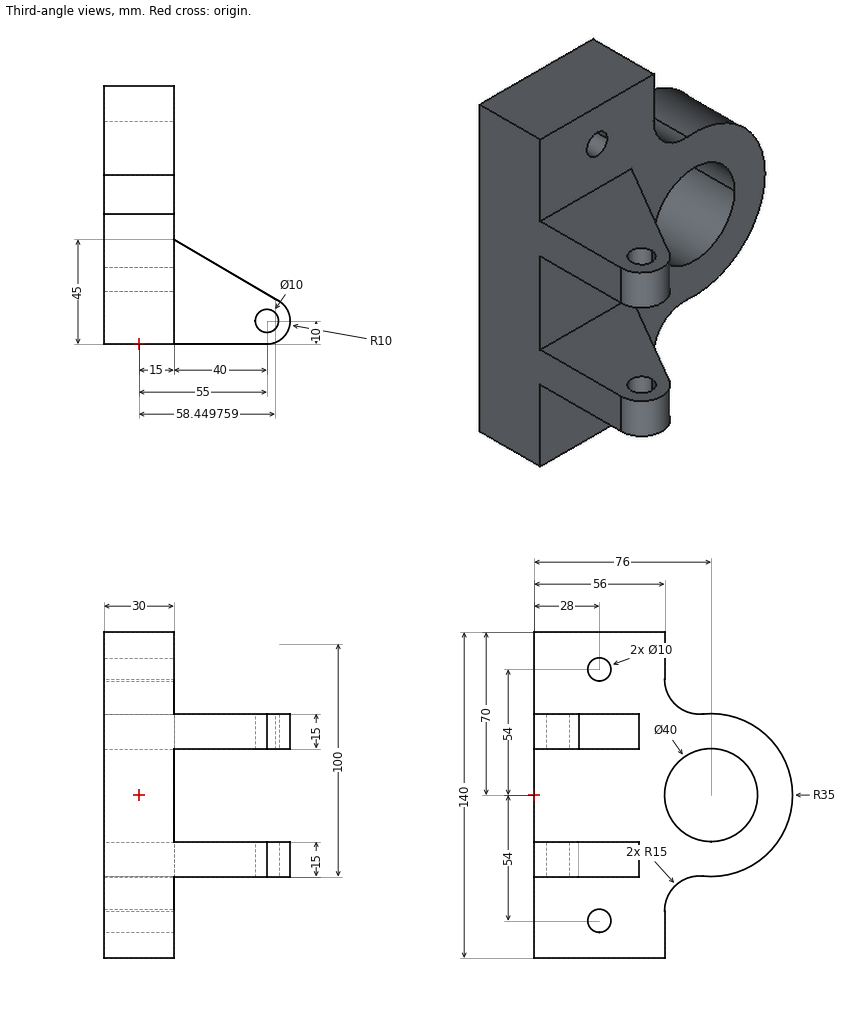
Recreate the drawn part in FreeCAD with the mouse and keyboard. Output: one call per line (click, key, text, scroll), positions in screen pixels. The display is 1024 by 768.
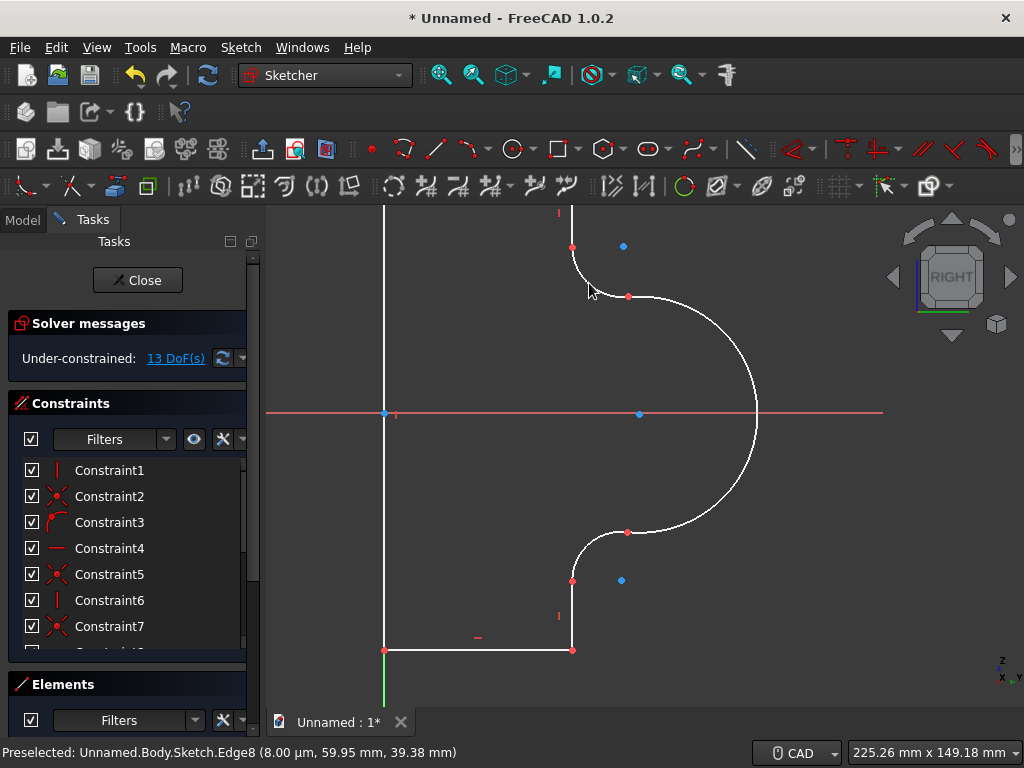
click(572, 234)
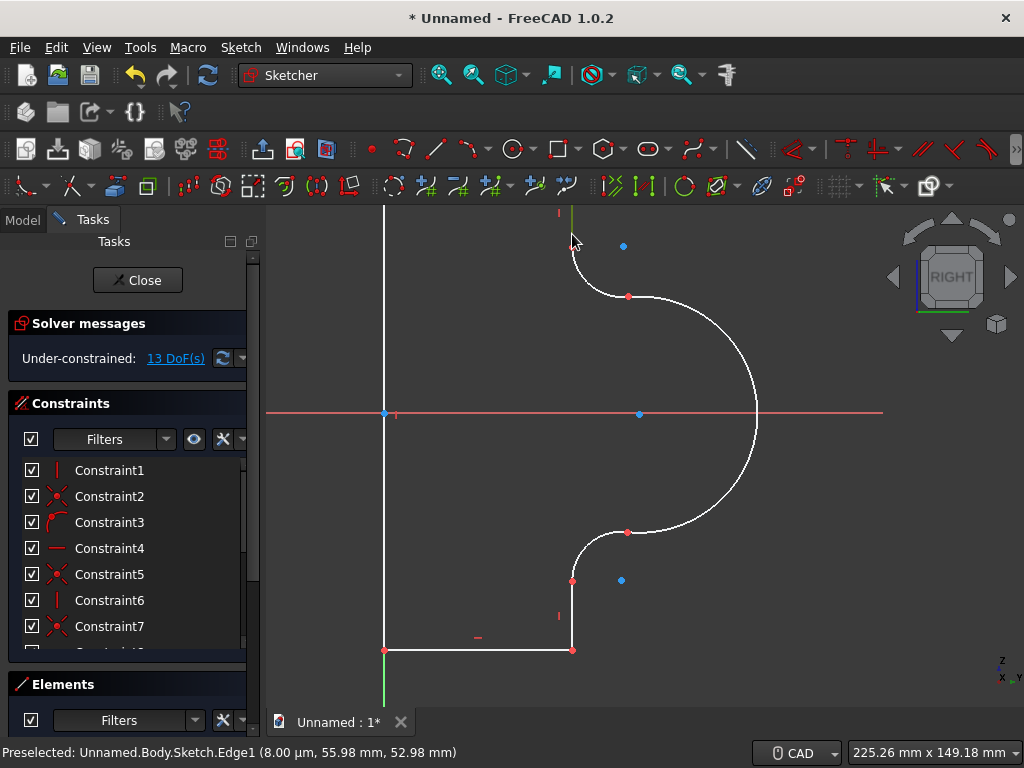
click(579, 271)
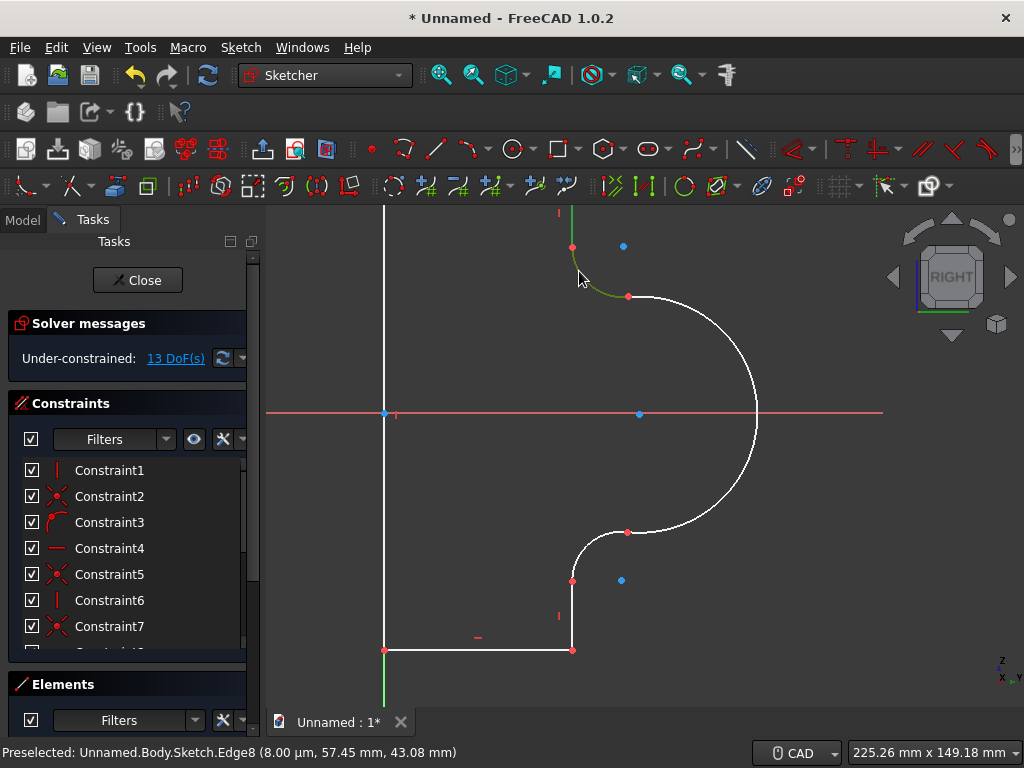
key(t)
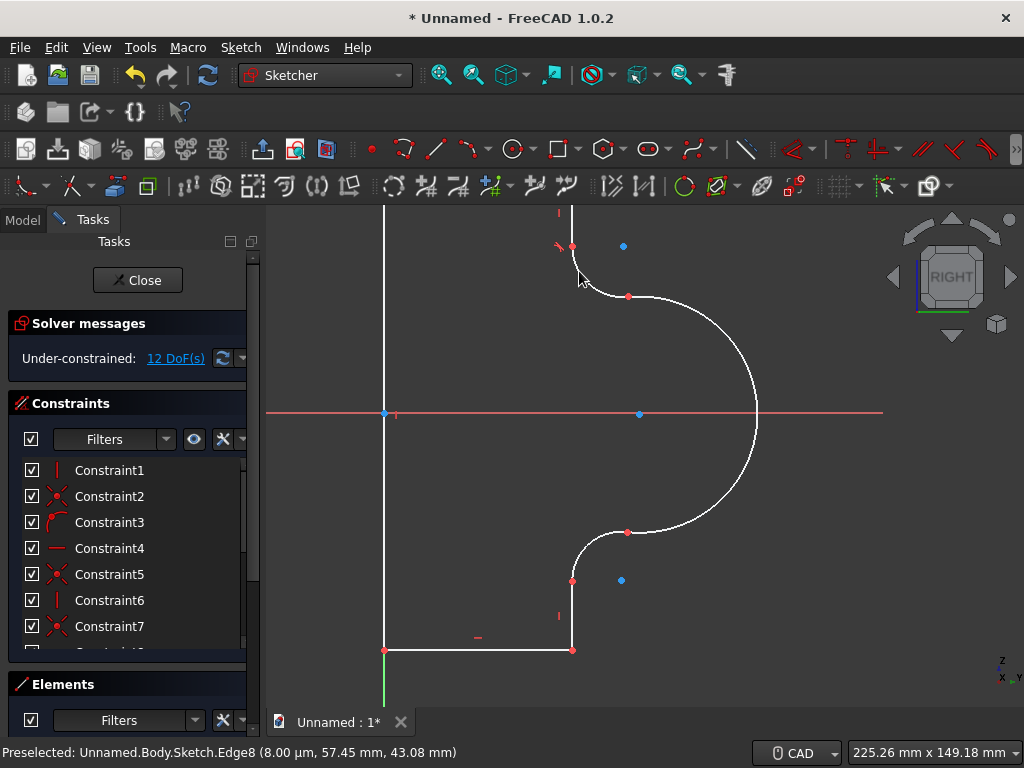
click(572, 629)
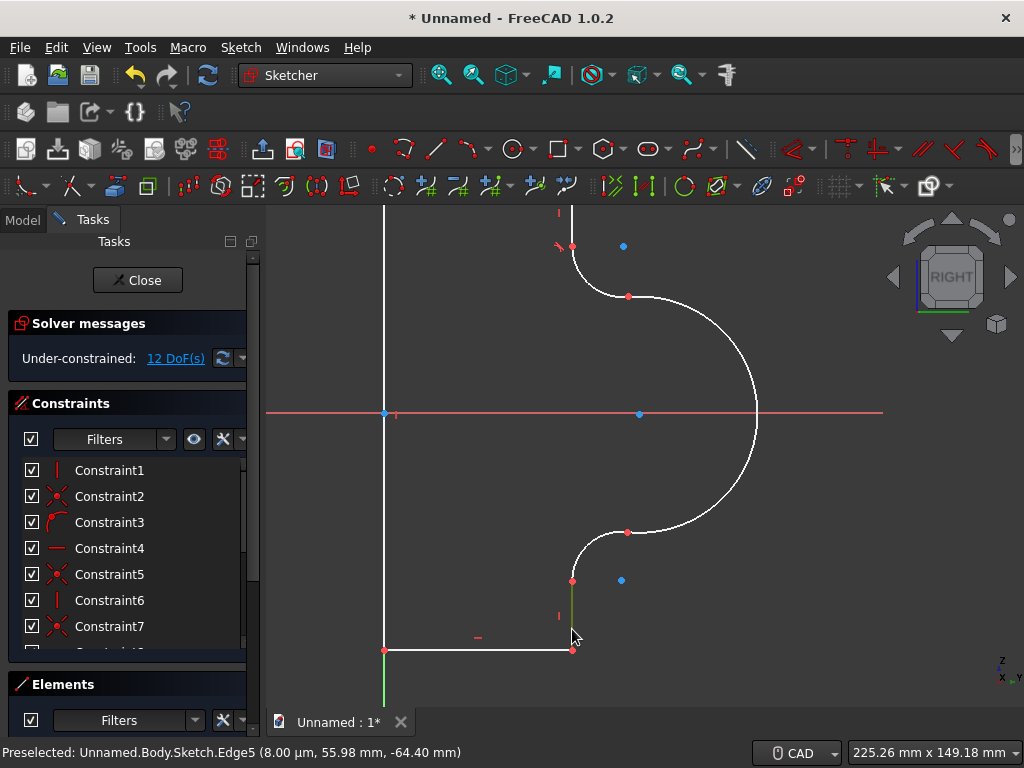
click(603, 535)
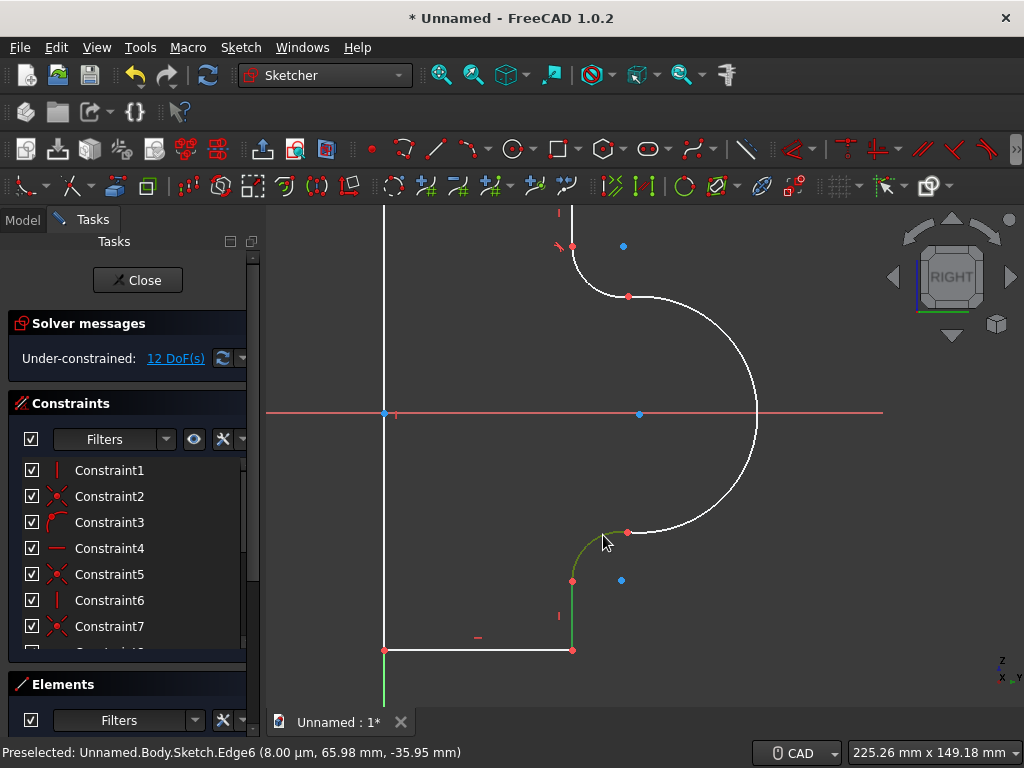
click(988, 150)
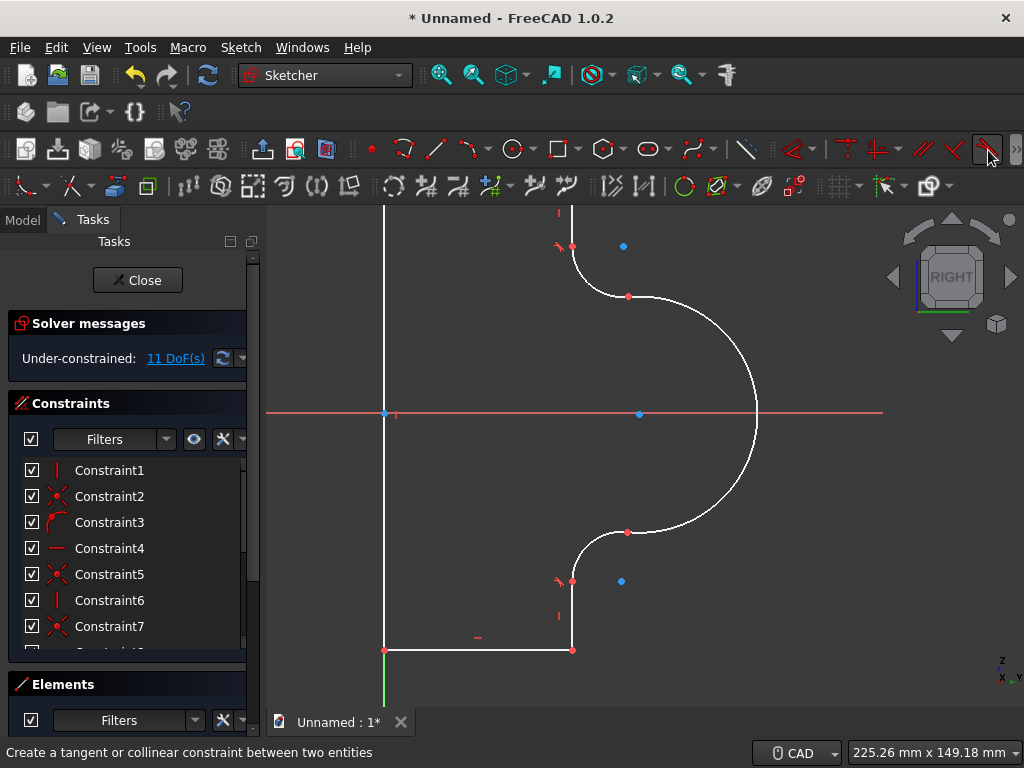
click(603, 536)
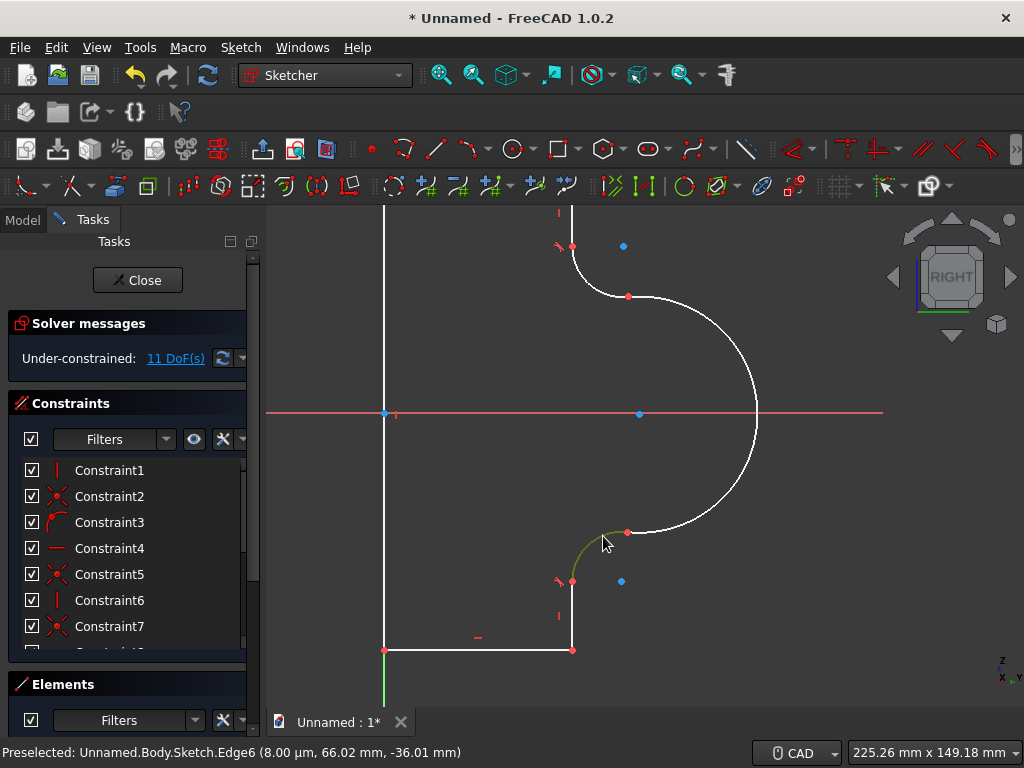
click(732, 488)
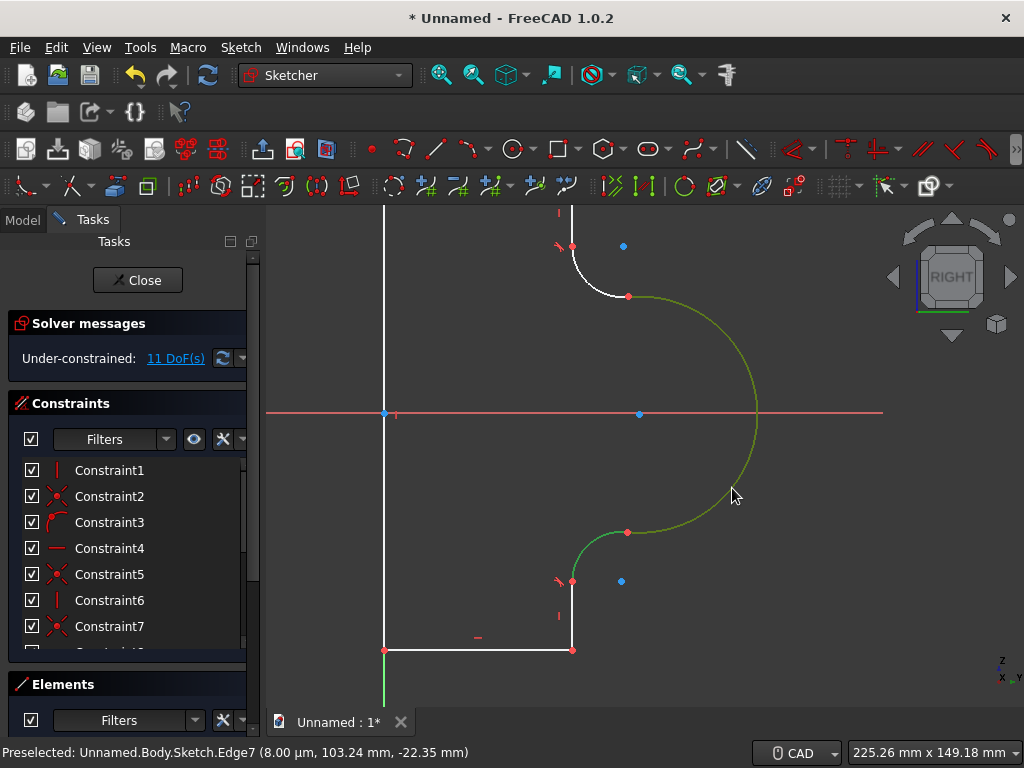
click(988, 150)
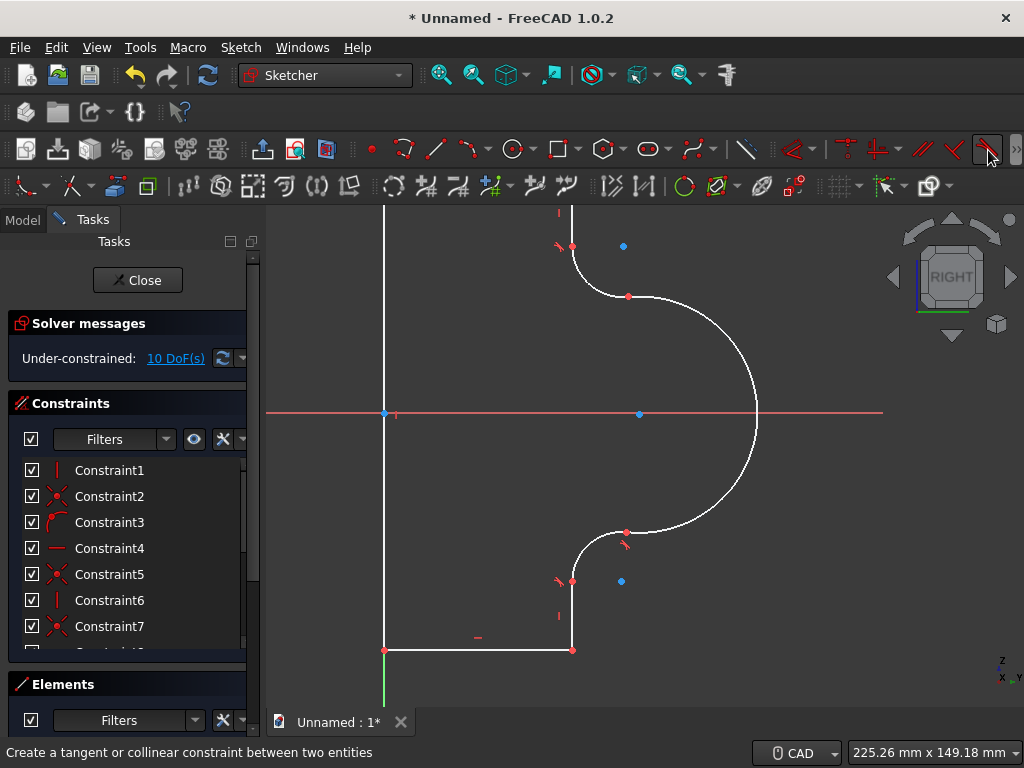
click(732, 488)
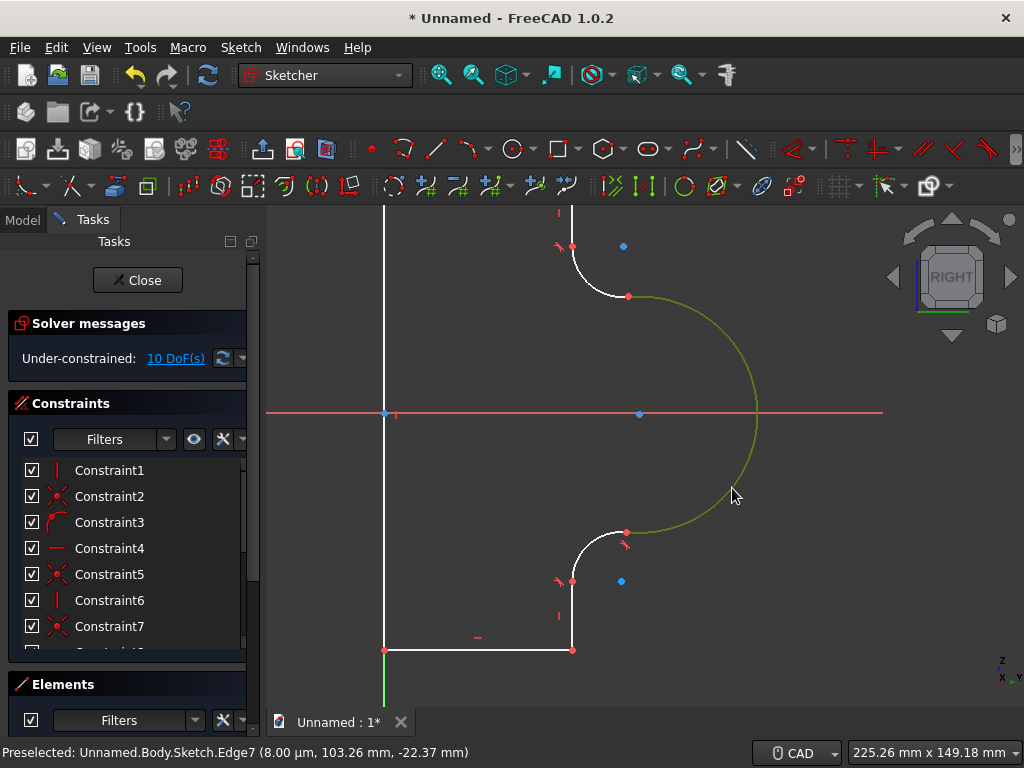
click(579, 271)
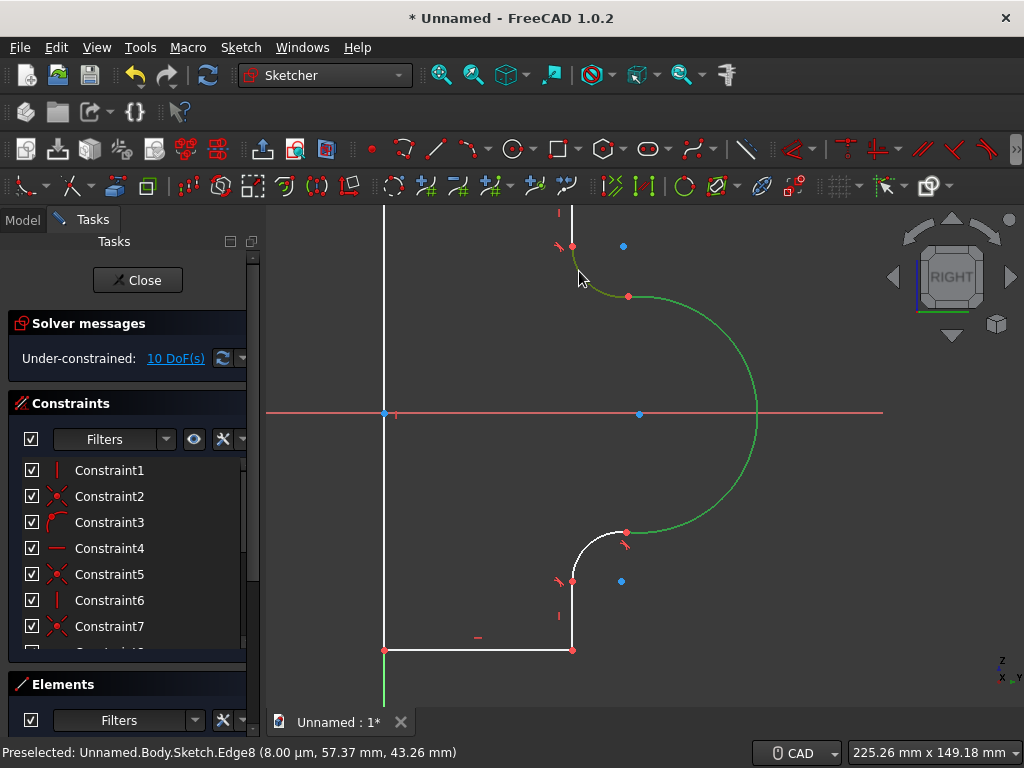
key(t)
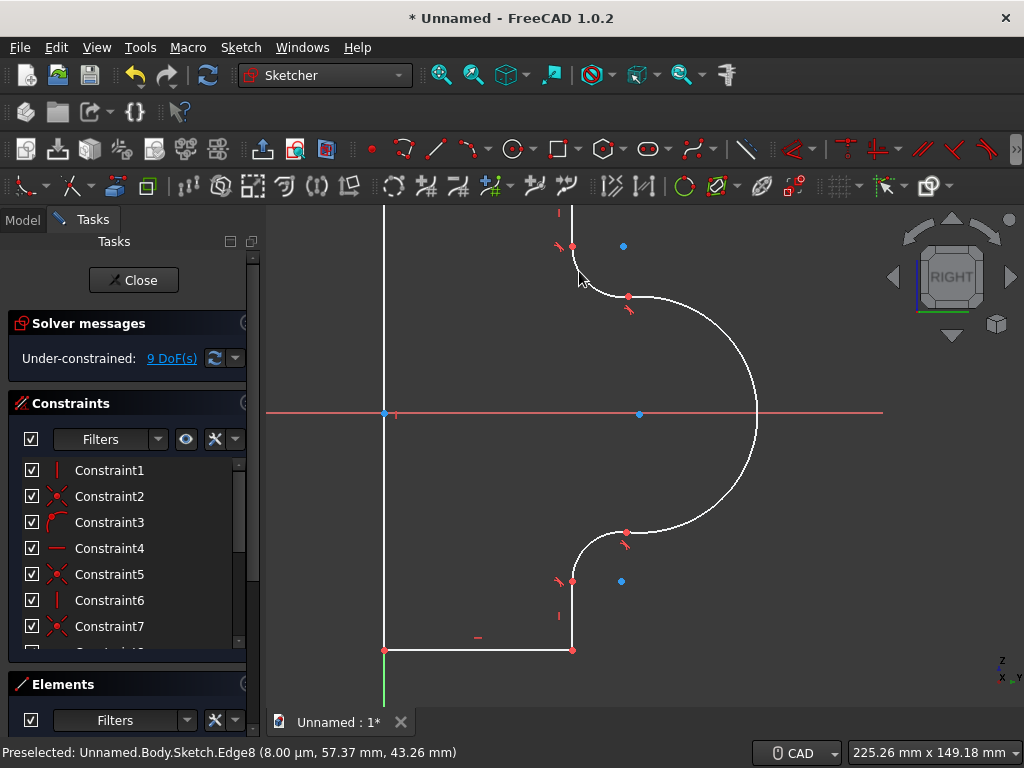
click(603, 536)